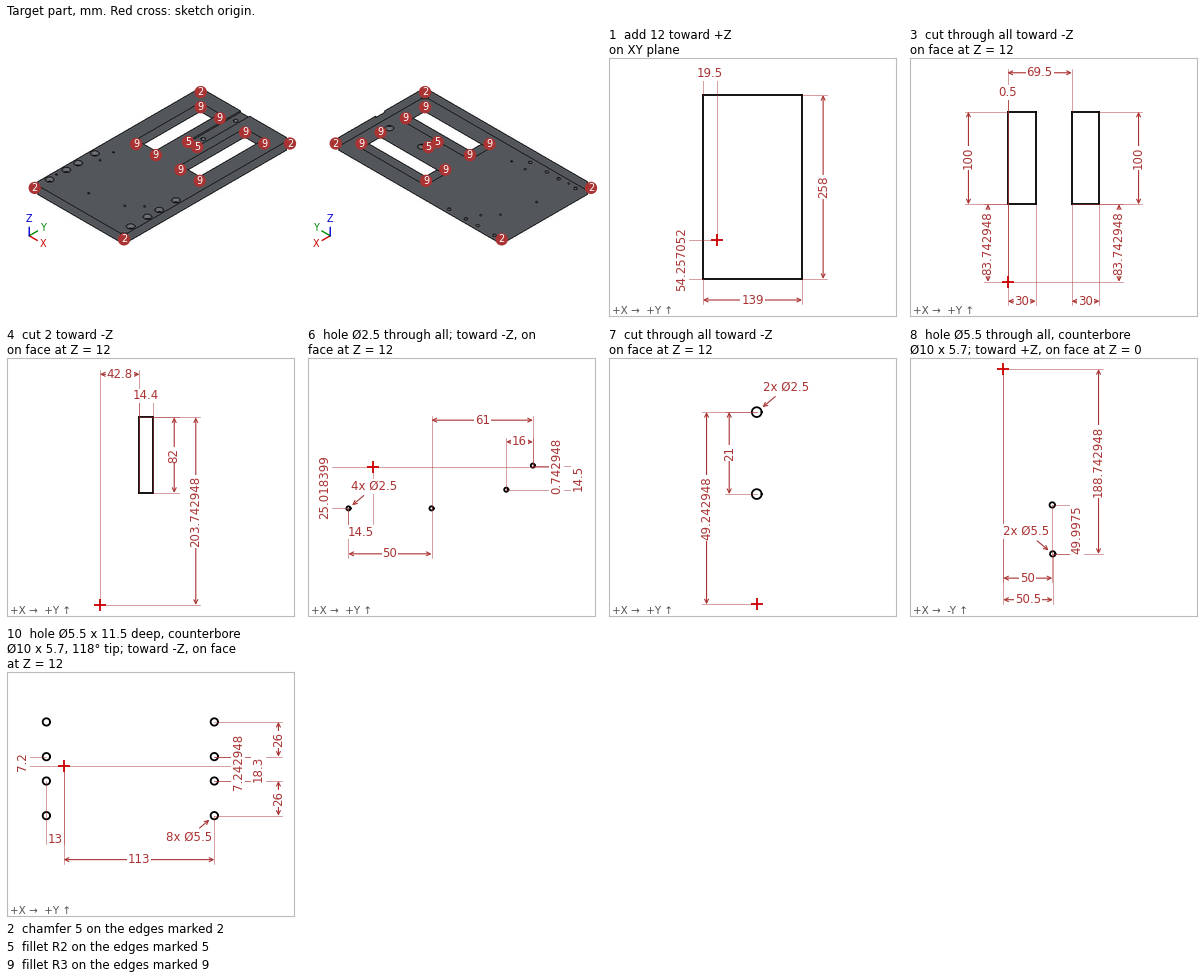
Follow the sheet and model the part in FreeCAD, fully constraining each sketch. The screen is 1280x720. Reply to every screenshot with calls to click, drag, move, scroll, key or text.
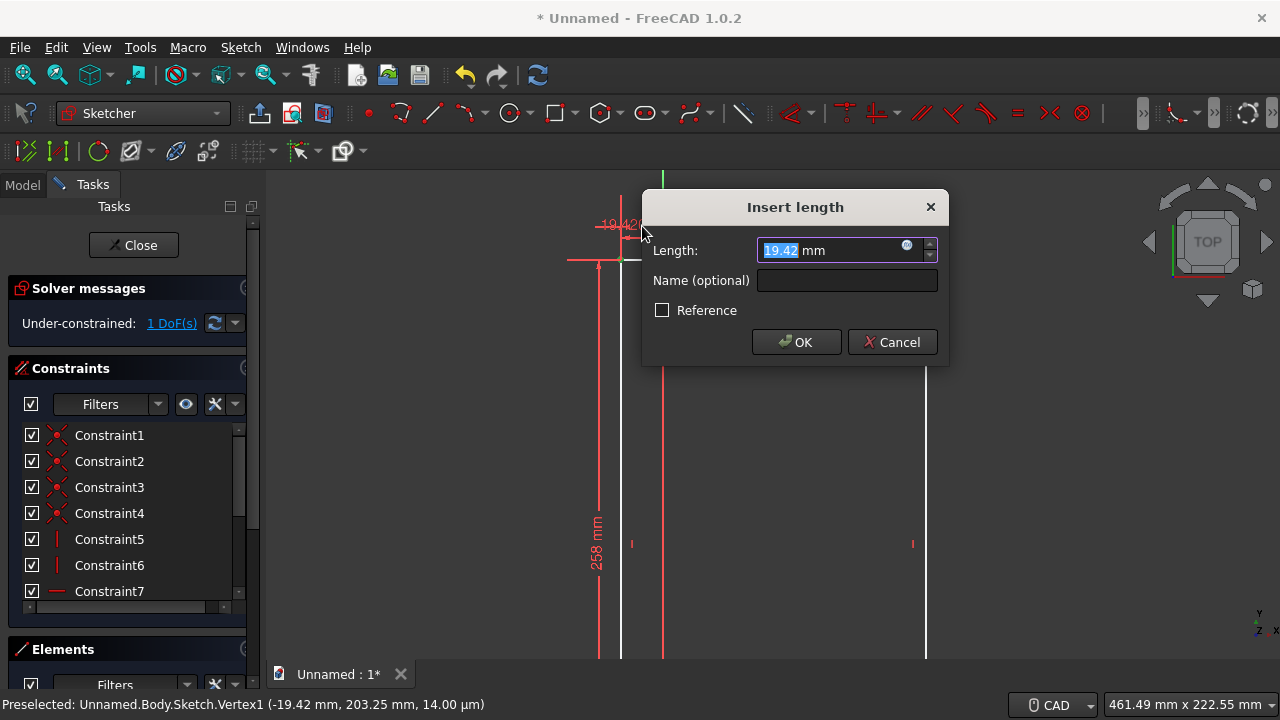
text(19.5)
key(Return)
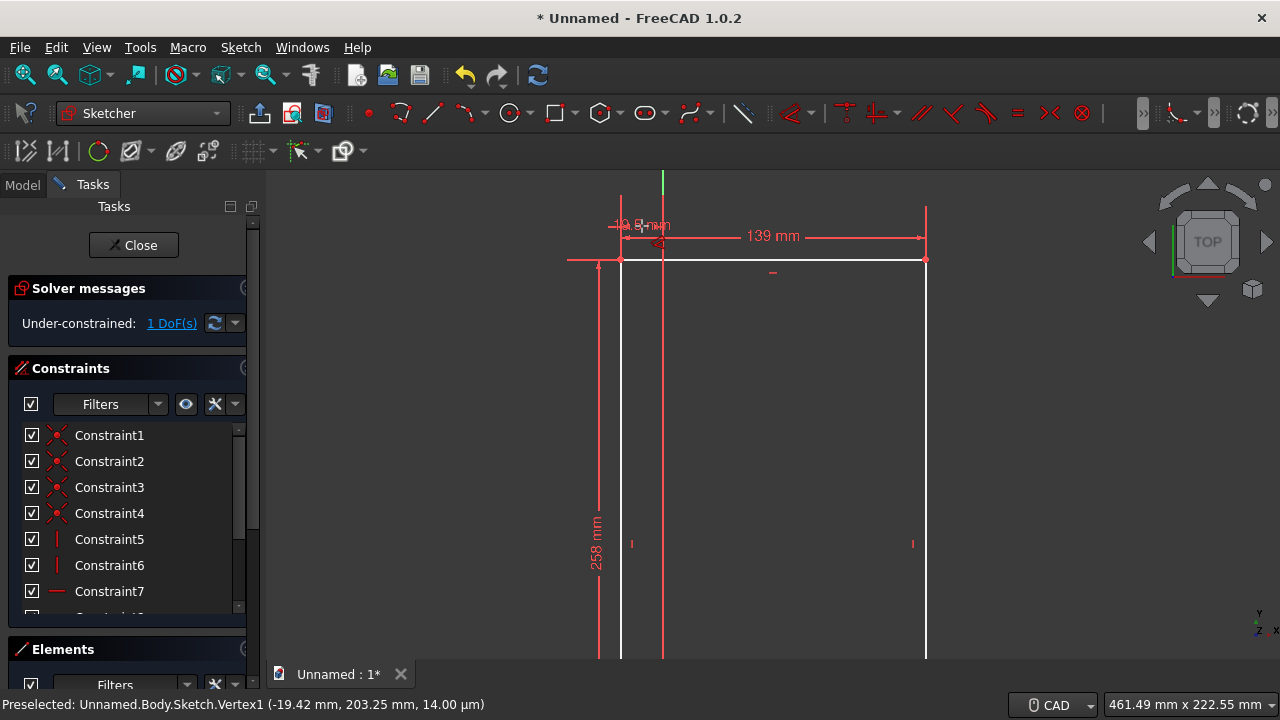
scroll(621, 259, down, 3)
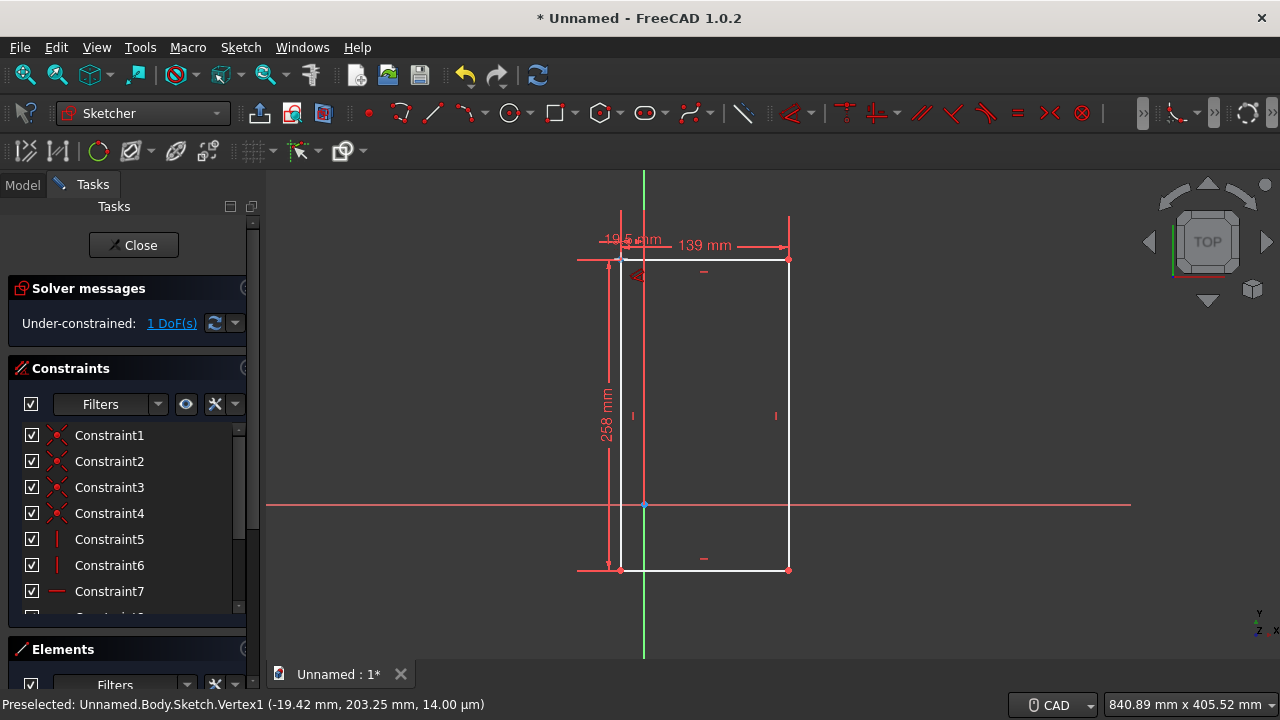
click(621, 571)
click(587, 538)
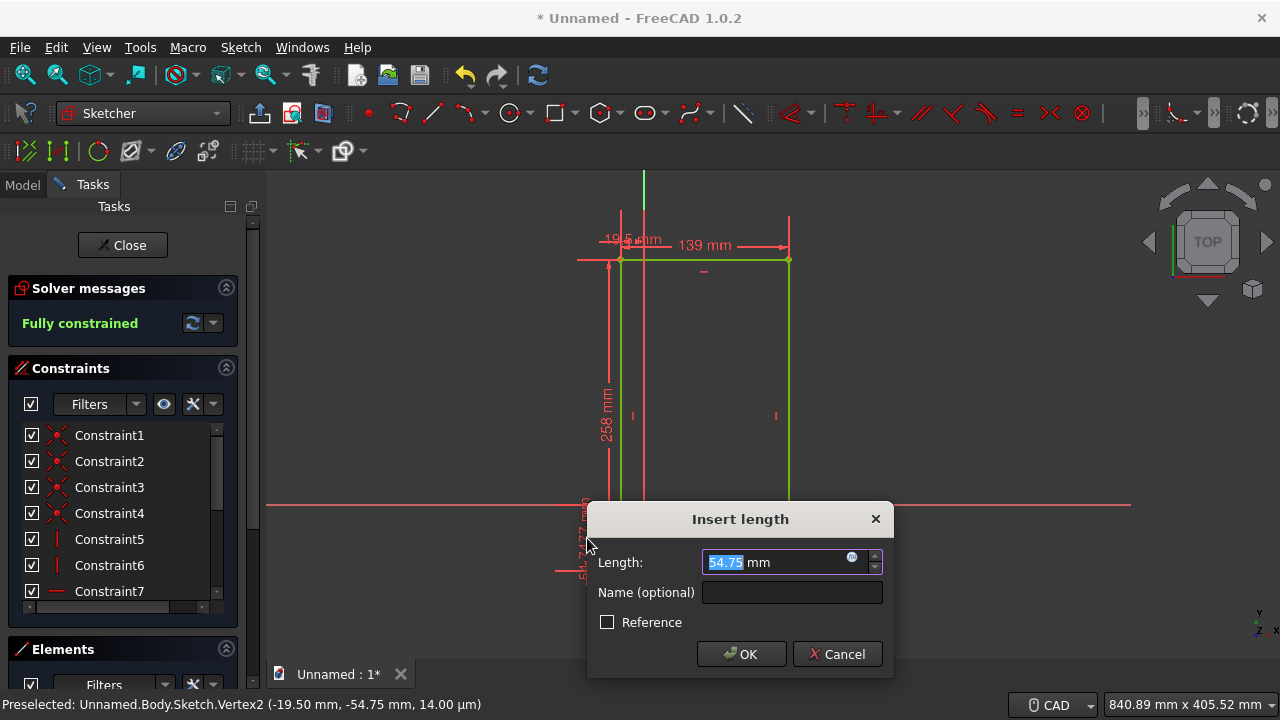
text(54.257052)
key(Return)
key(Escape)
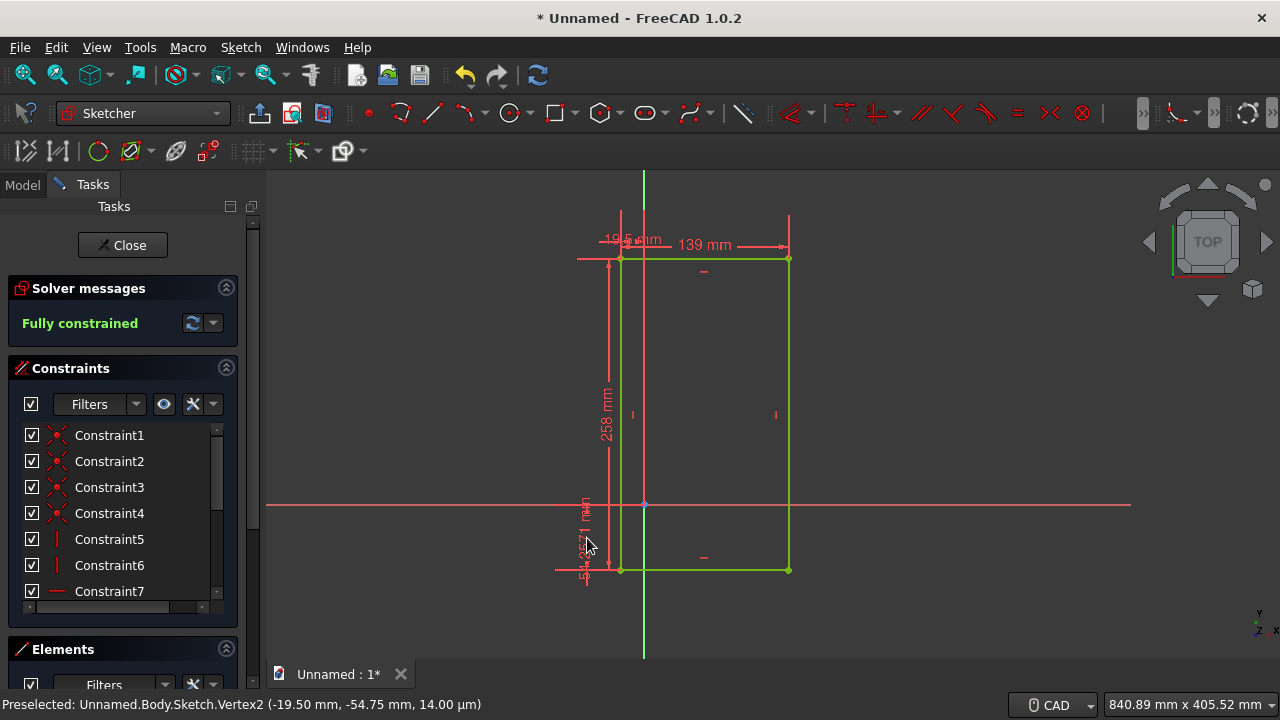
click(123, 245)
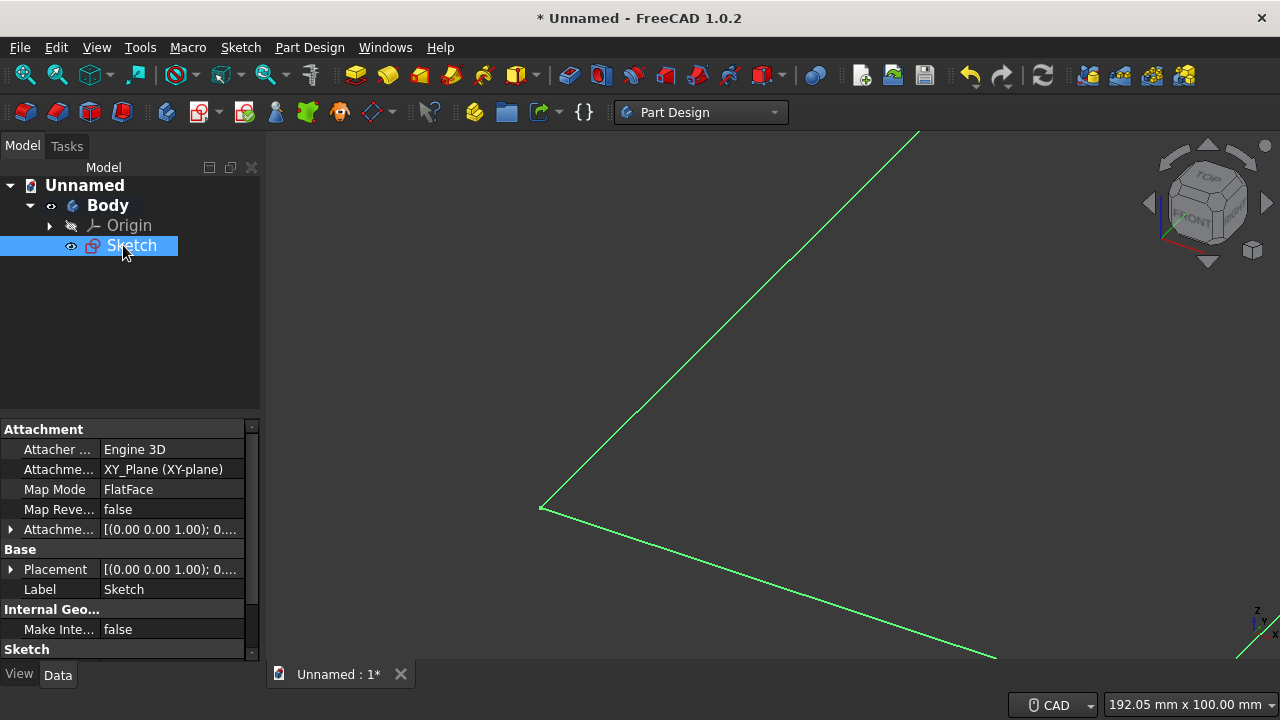
click(356, 76)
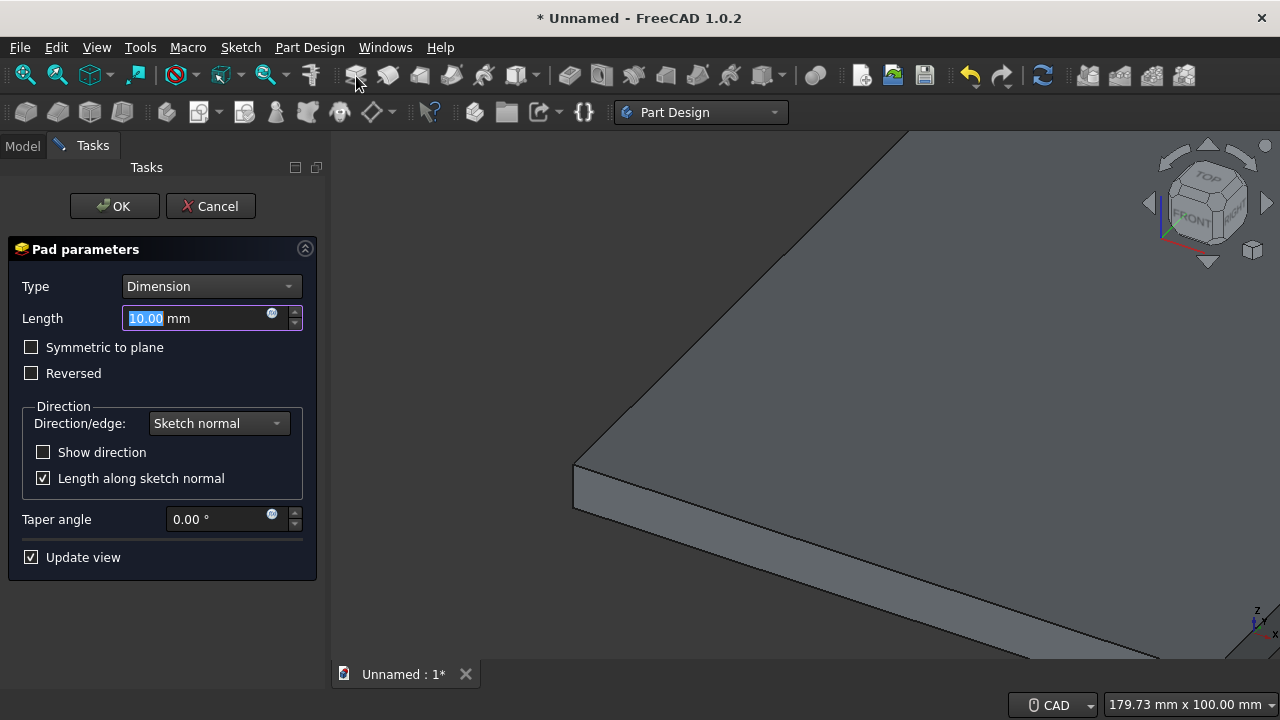
text(12)
key(Tab)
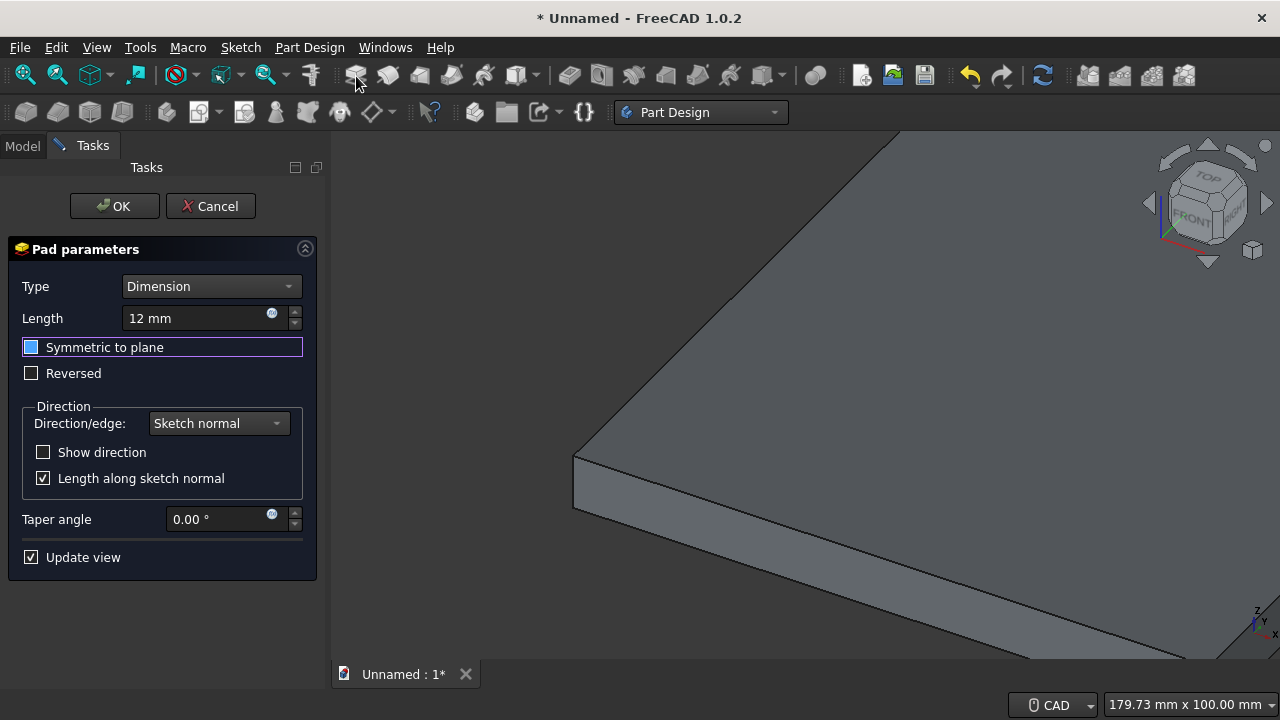
click(115, 206)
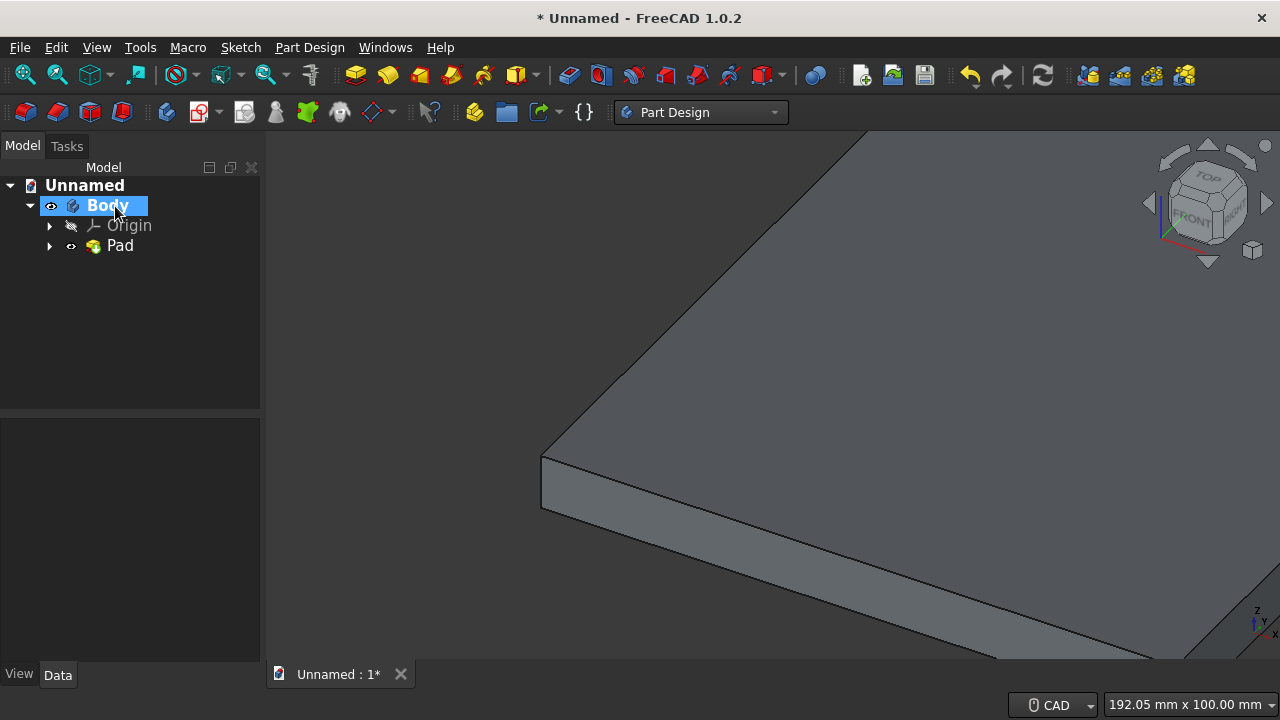
key(v)
key(f)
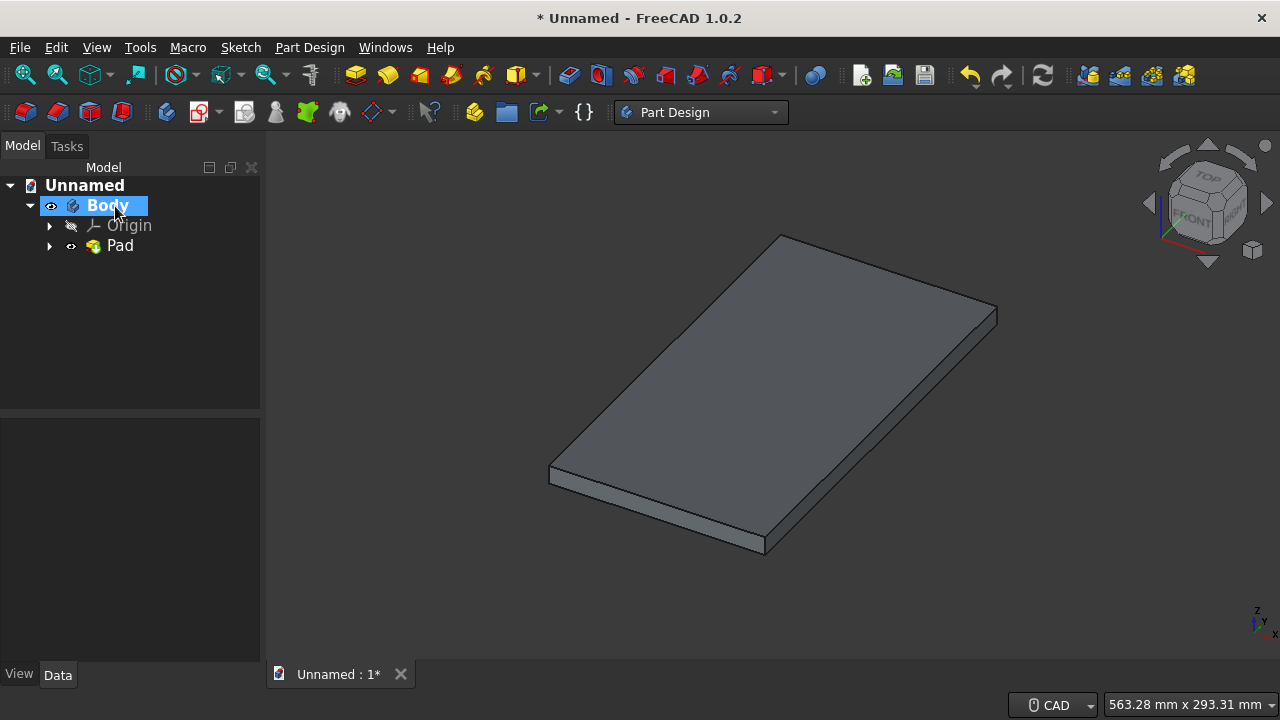
click(765, 545)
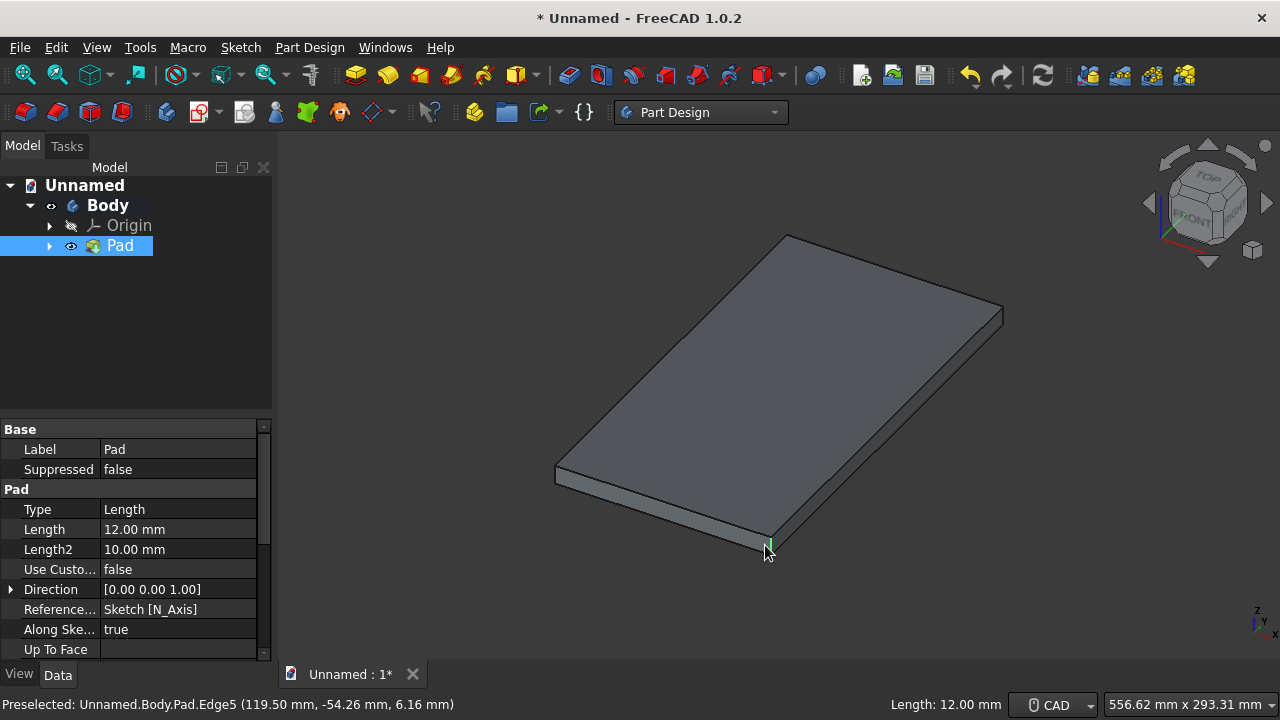
scroll(555, 473, up, 4)